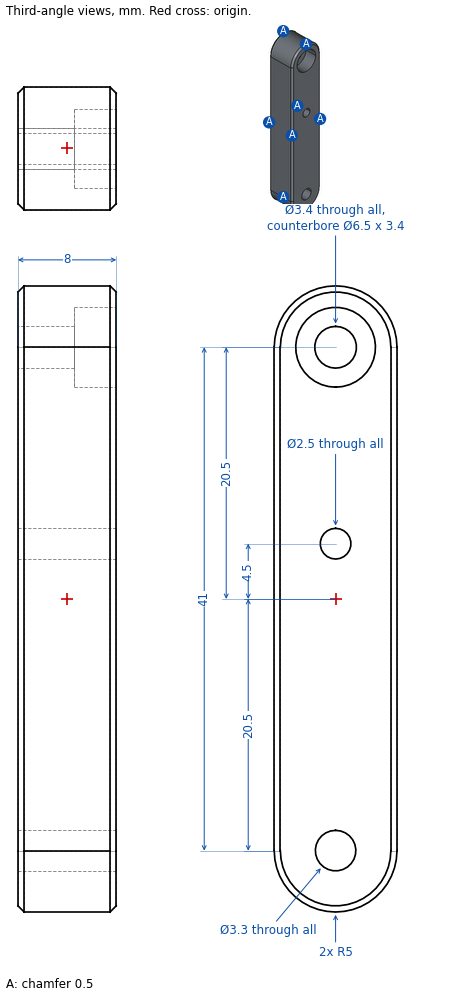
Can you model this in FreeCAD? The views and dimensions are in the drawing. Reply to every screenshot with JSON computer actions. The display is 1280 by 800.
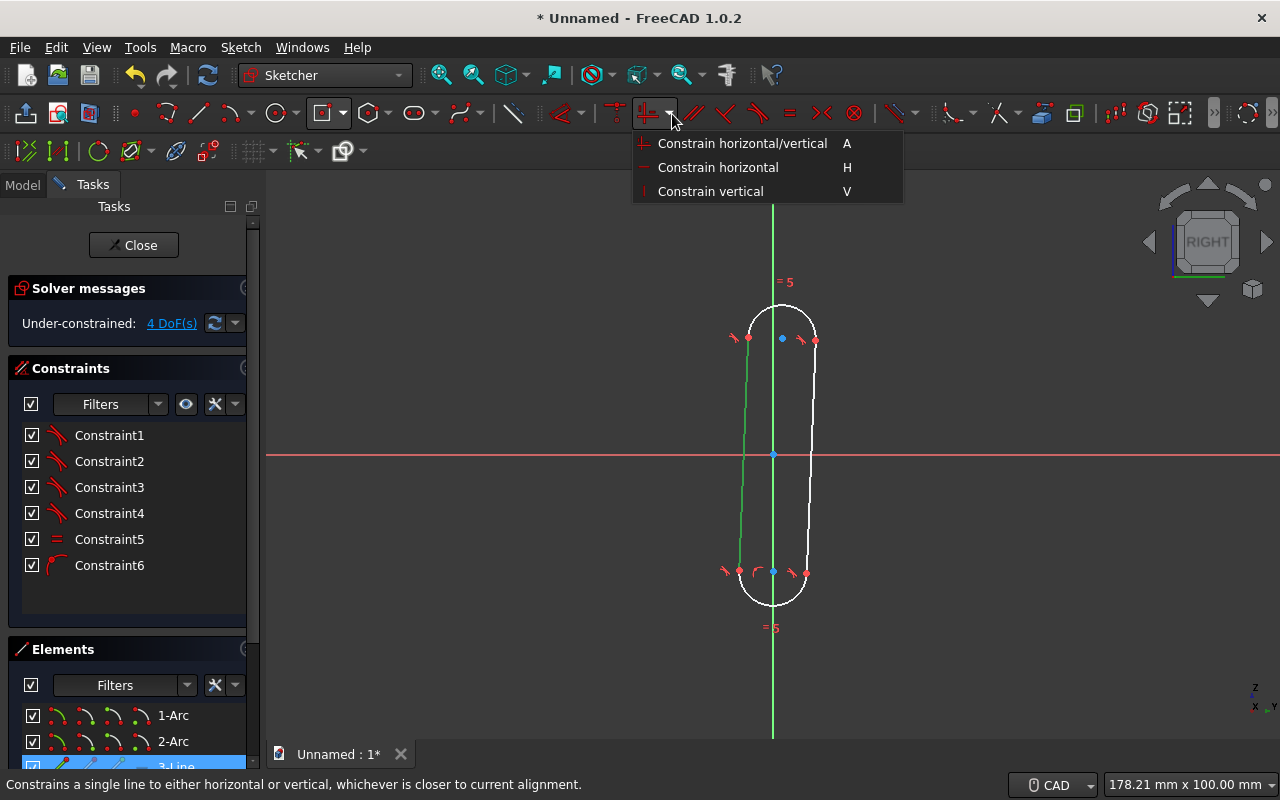
{"action": "left_click", "coordinate": [768, 191]}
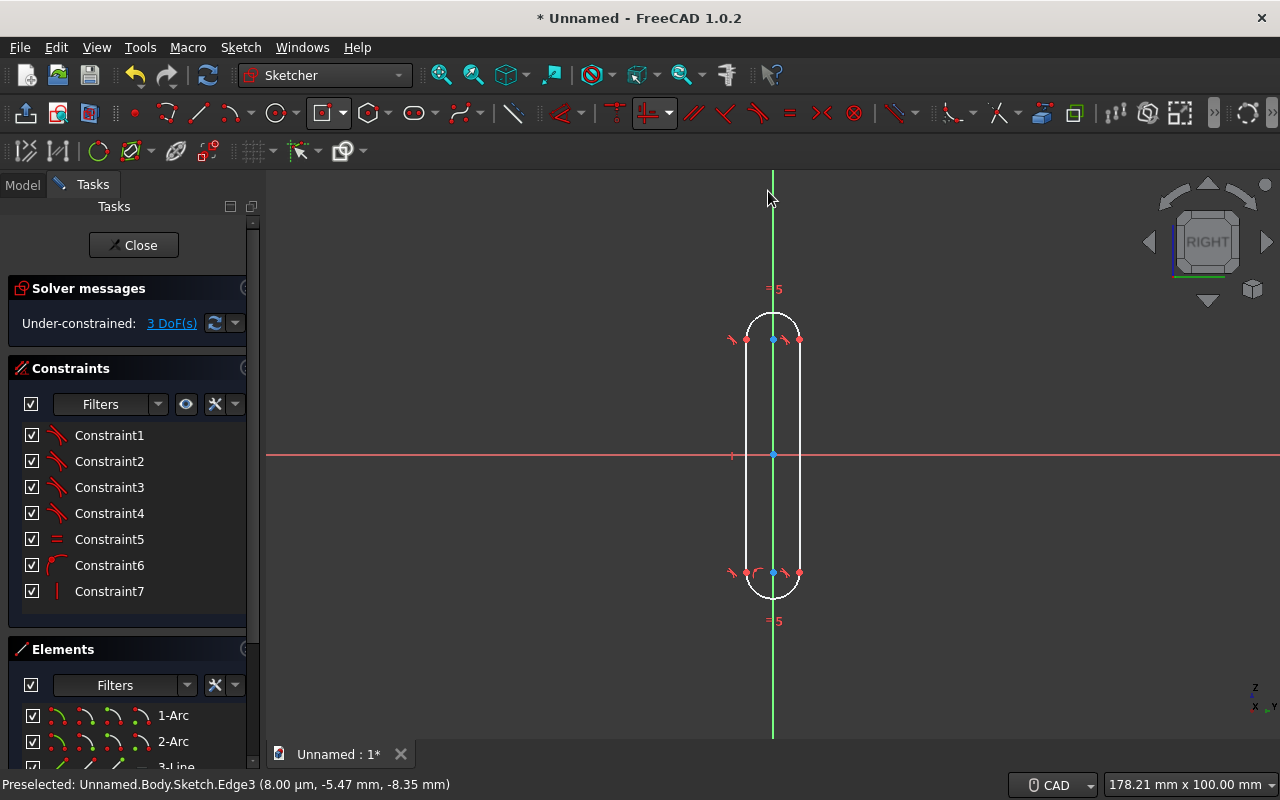
{"action": "key", "text": "d"}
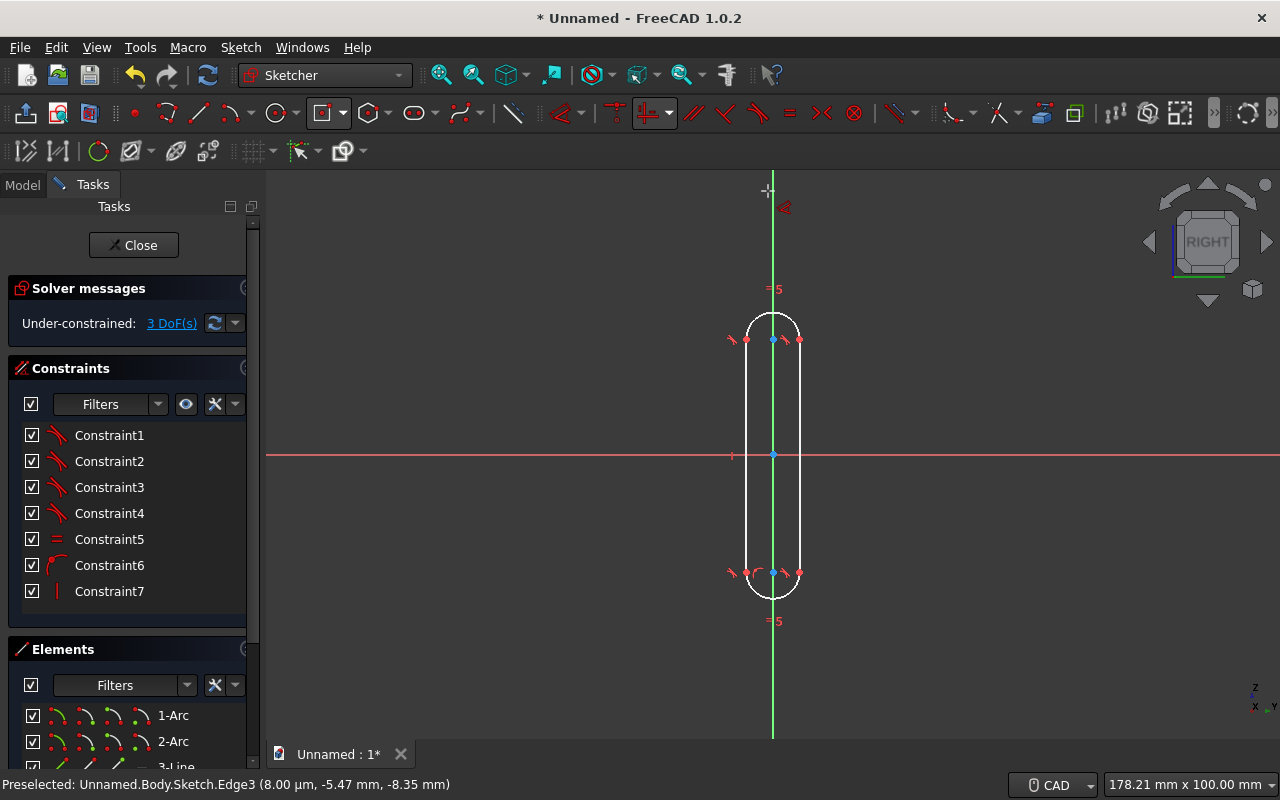
{"action": "scroll", "coordinate": [757, 594], "scroll_direction": "up", "scroll_amount": 2}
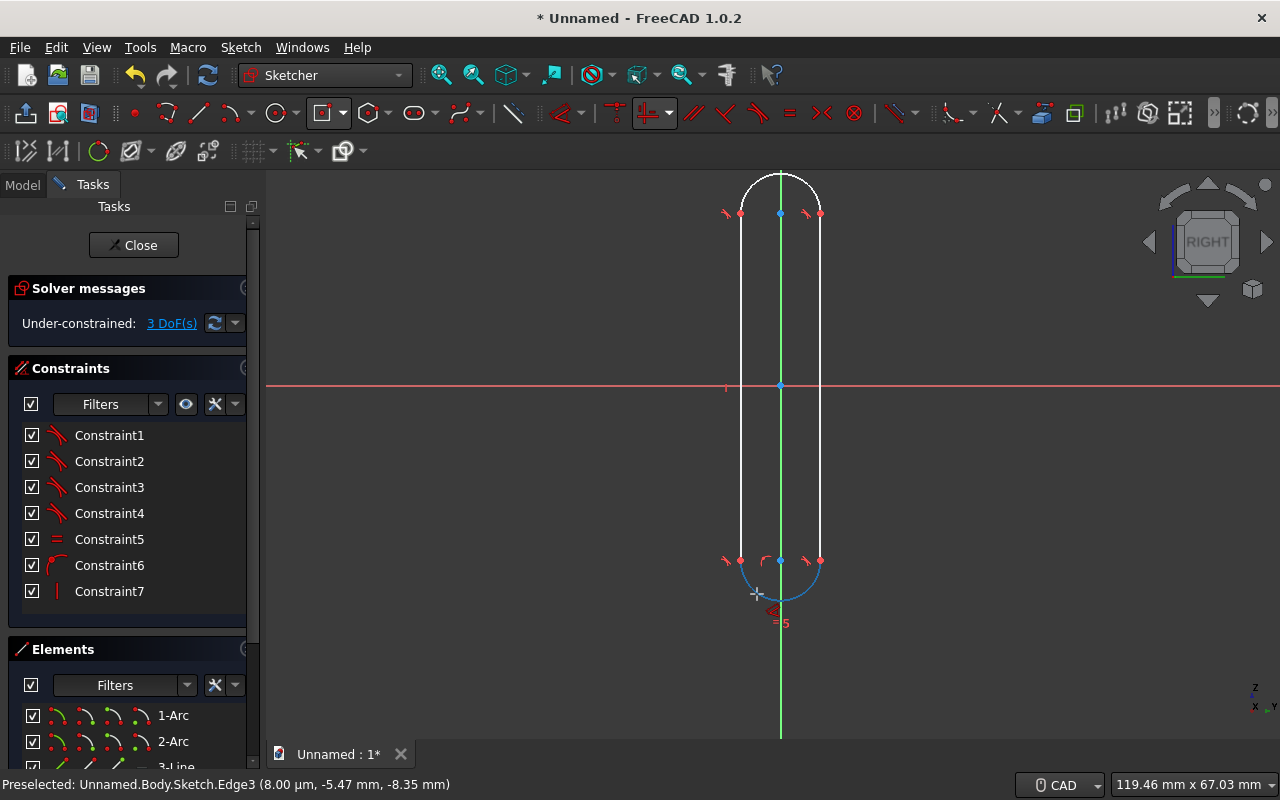
{"action": "left_click", "coordinate": [757, 593]}
{"action": "left_click", "coordinate": [738, 619]}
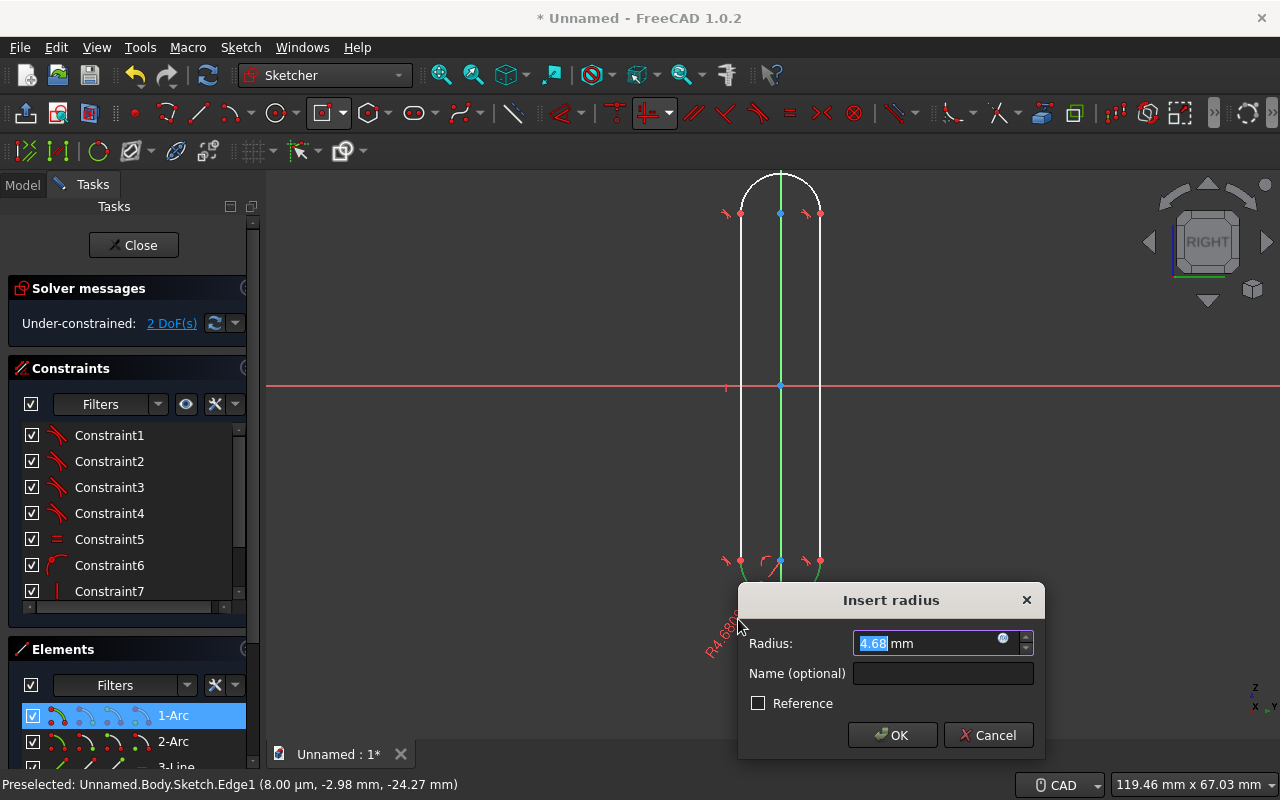
{"action": "type", "text": "5"}
{"action": "key", "text": "Return"}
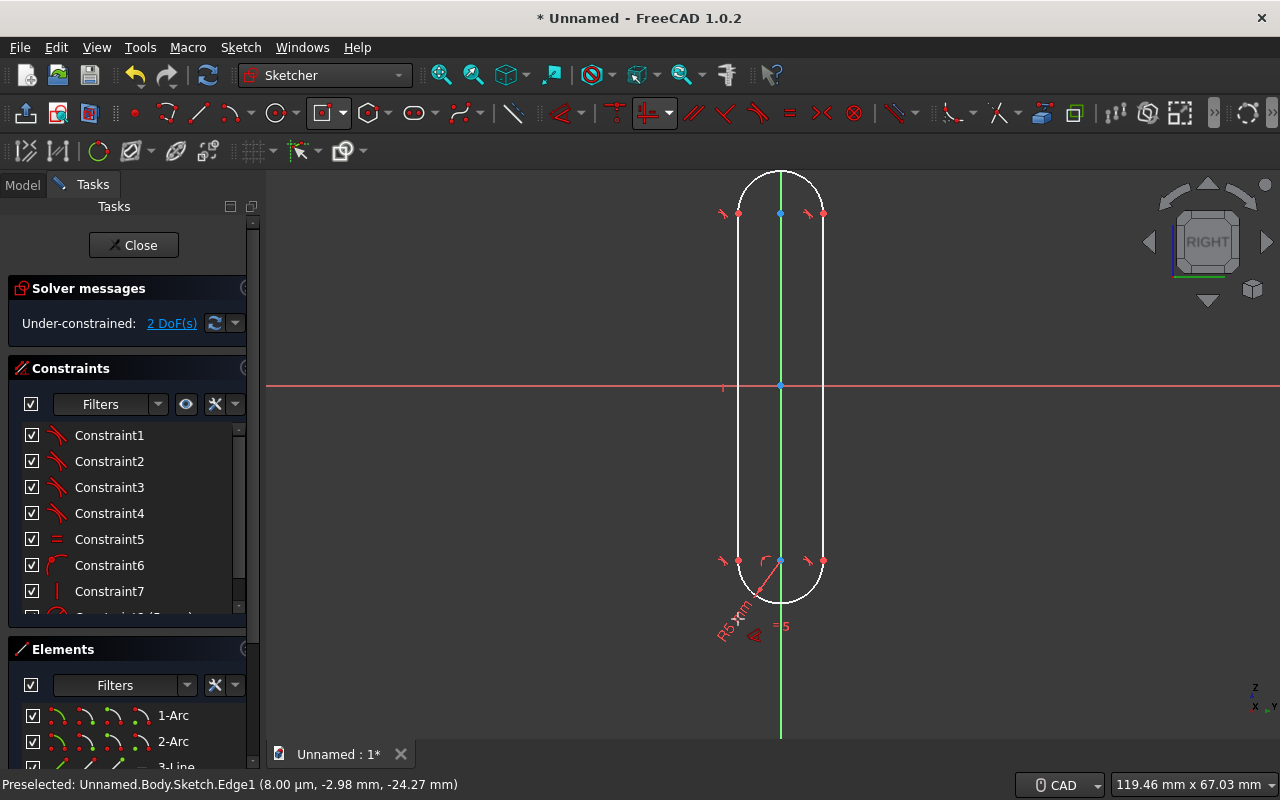
{"action": "left_click", "coordinate": [738, 457]}
{"action": "left_click", "coordinate": [704, 307]}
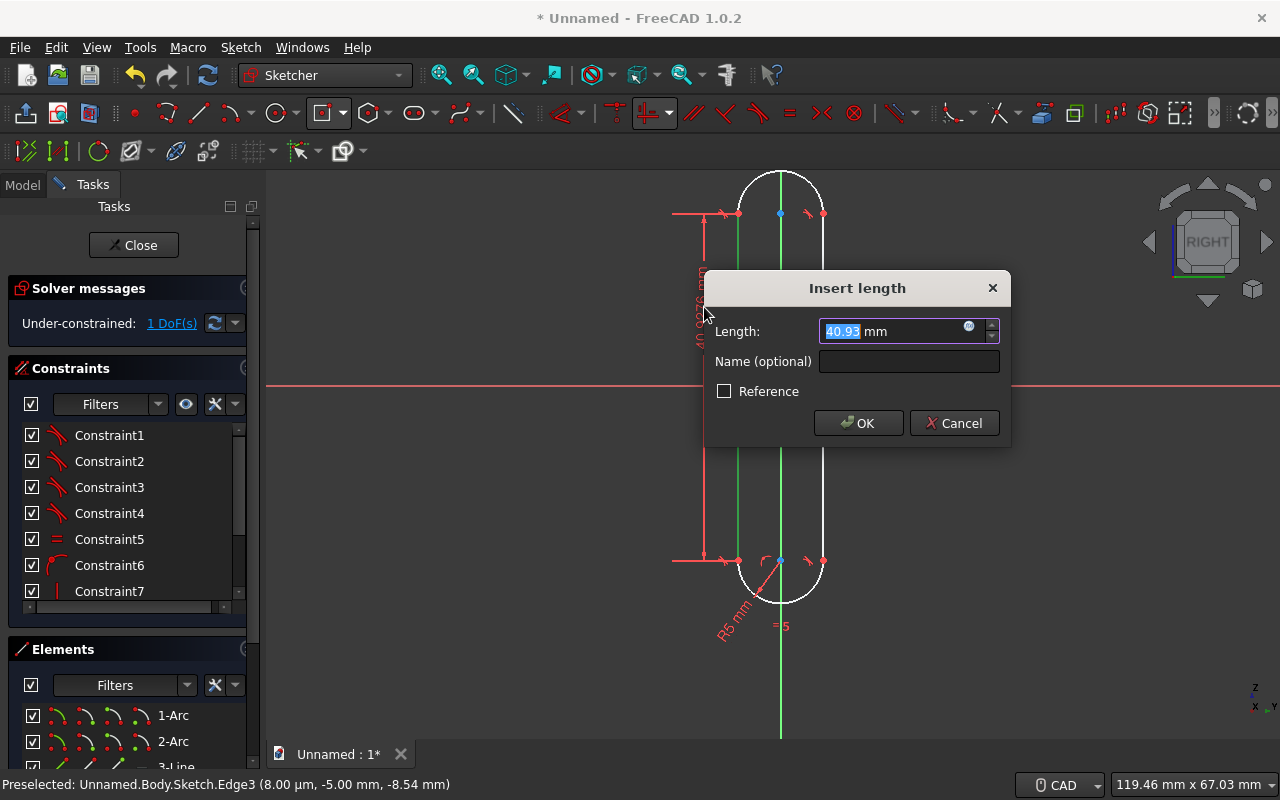
{"action": "type", "text": "41"}
{"action": "key", "text": "Return"}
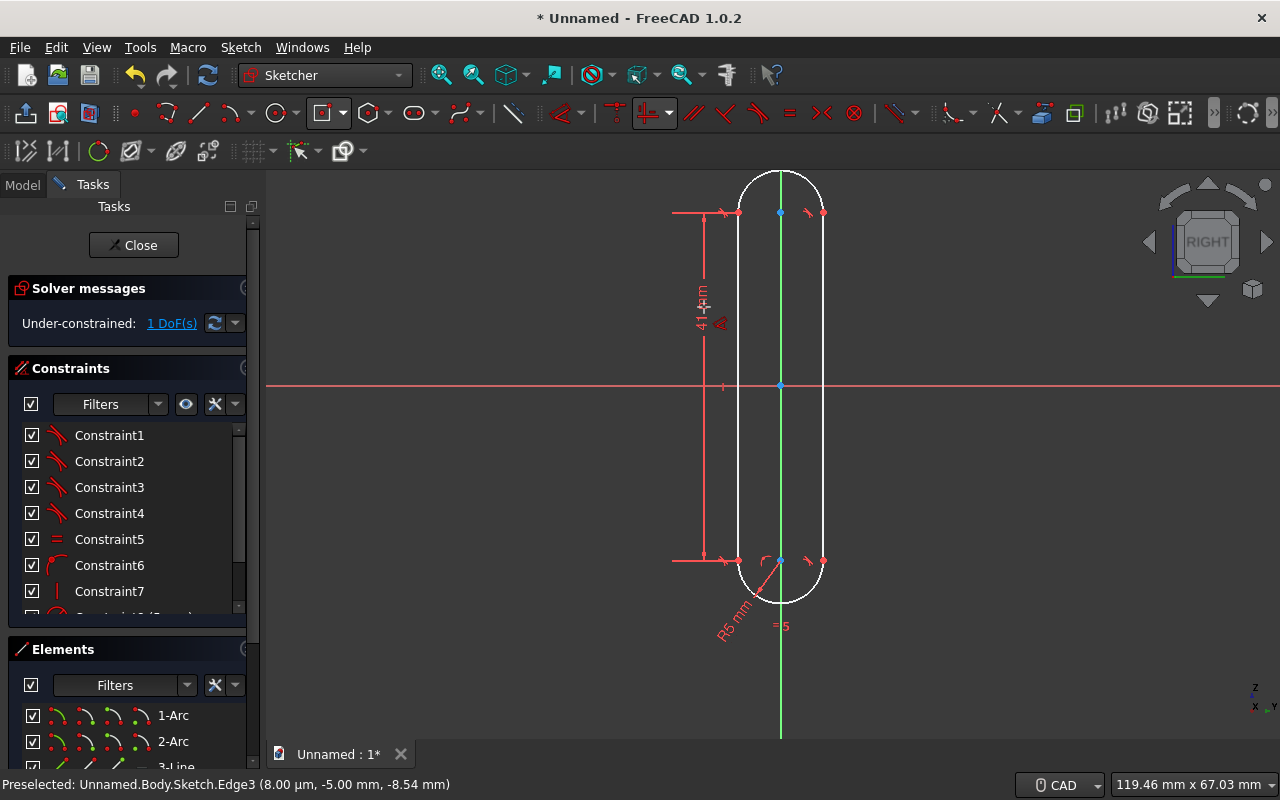
{"action": "left_click", "coordinate": [738, 561]}
{"action": "left_click", "coordinate": [704, 473]}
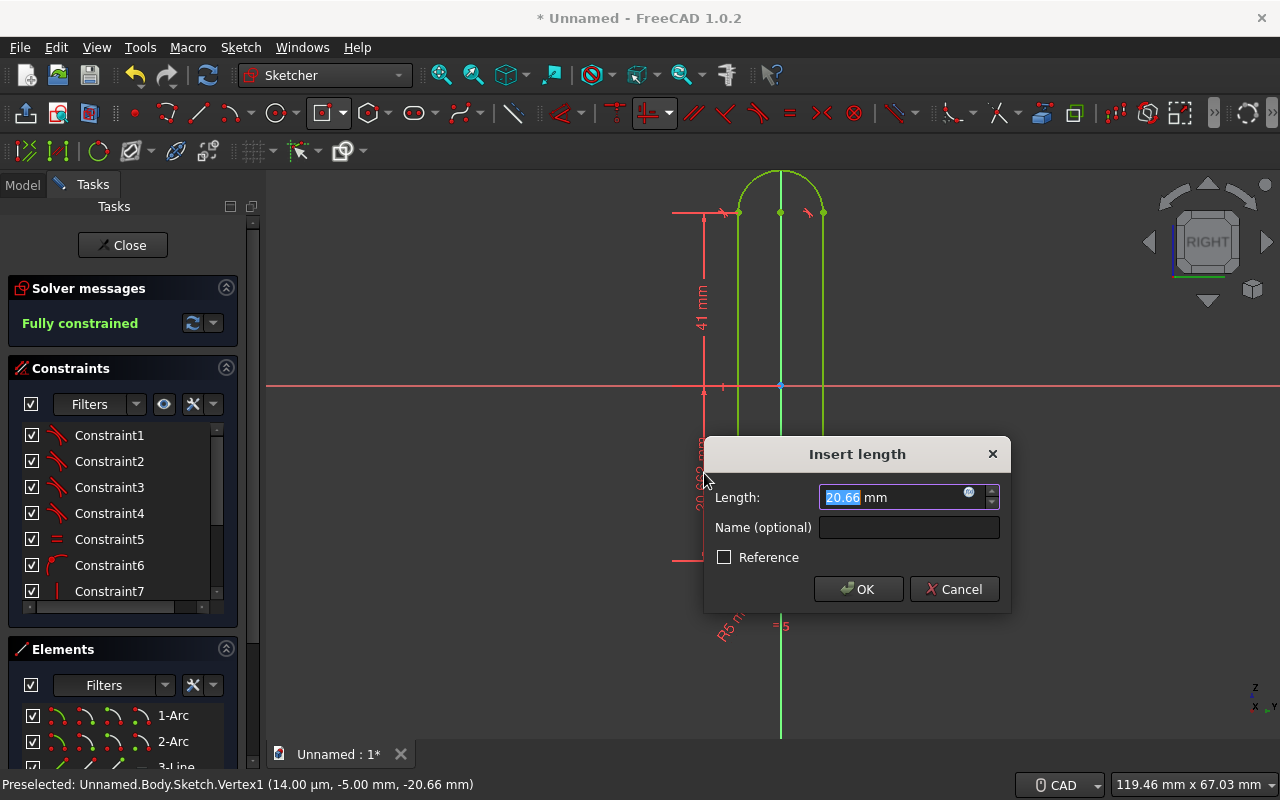
{"action": "type", "text": "20.5"}
{"action": "key", "text": "Return"}
{"action": "key", "text": "Escape"}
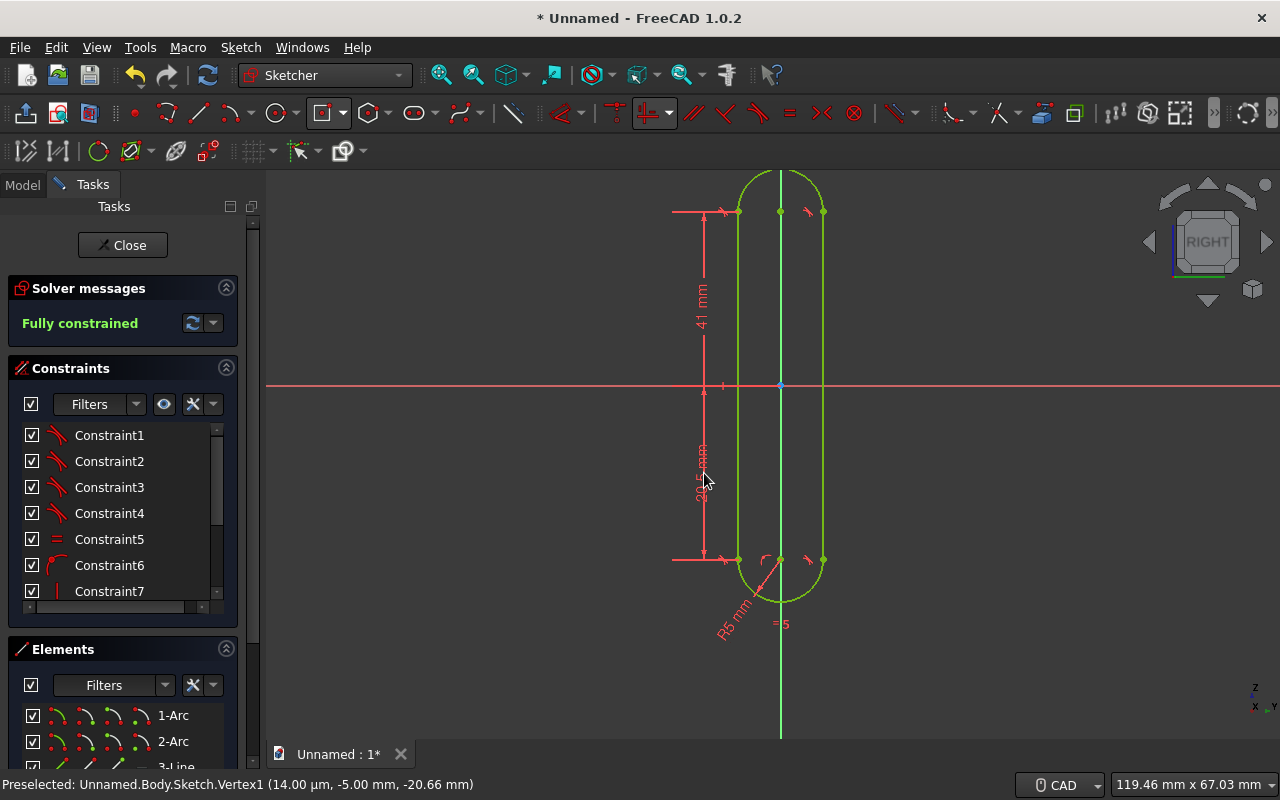
{"action": "left_click", "coordinate": [123, 245]}